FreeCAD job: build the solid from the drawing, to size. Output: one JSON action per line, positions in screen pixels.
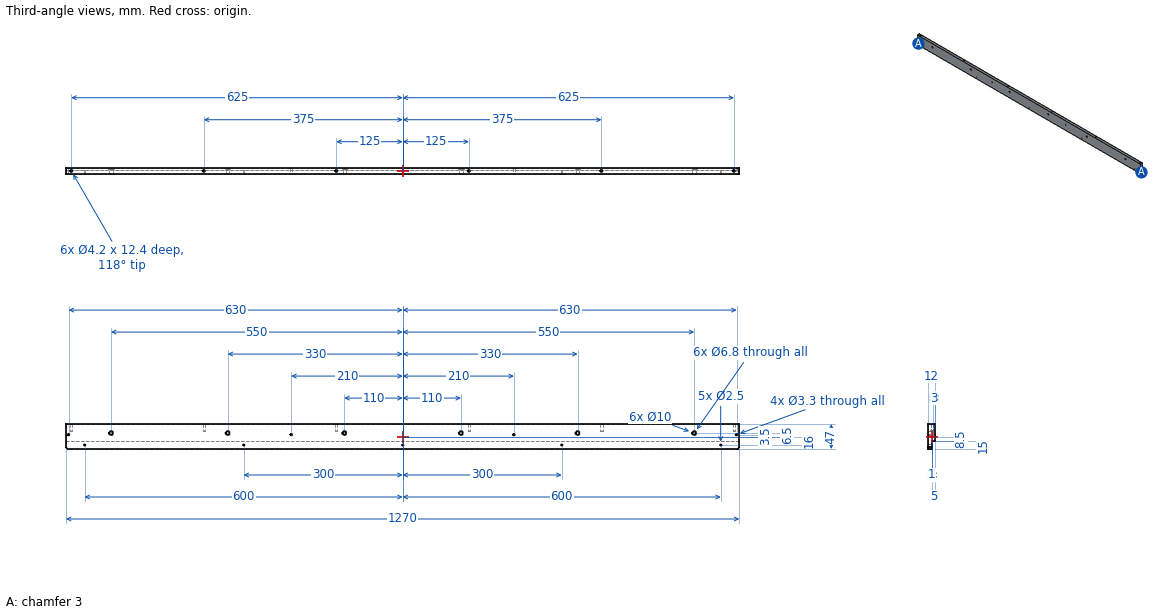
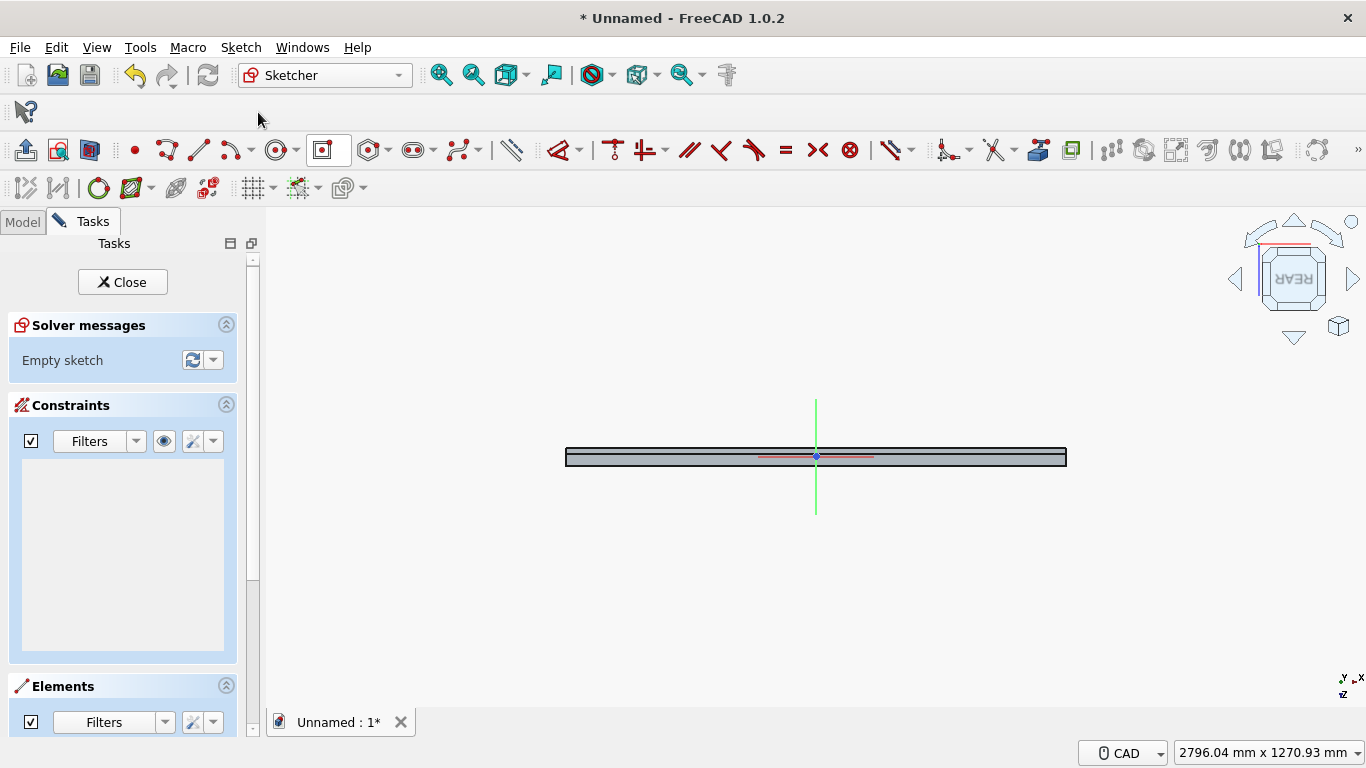
{"action": "left_click", "coordinate": [276, 150]}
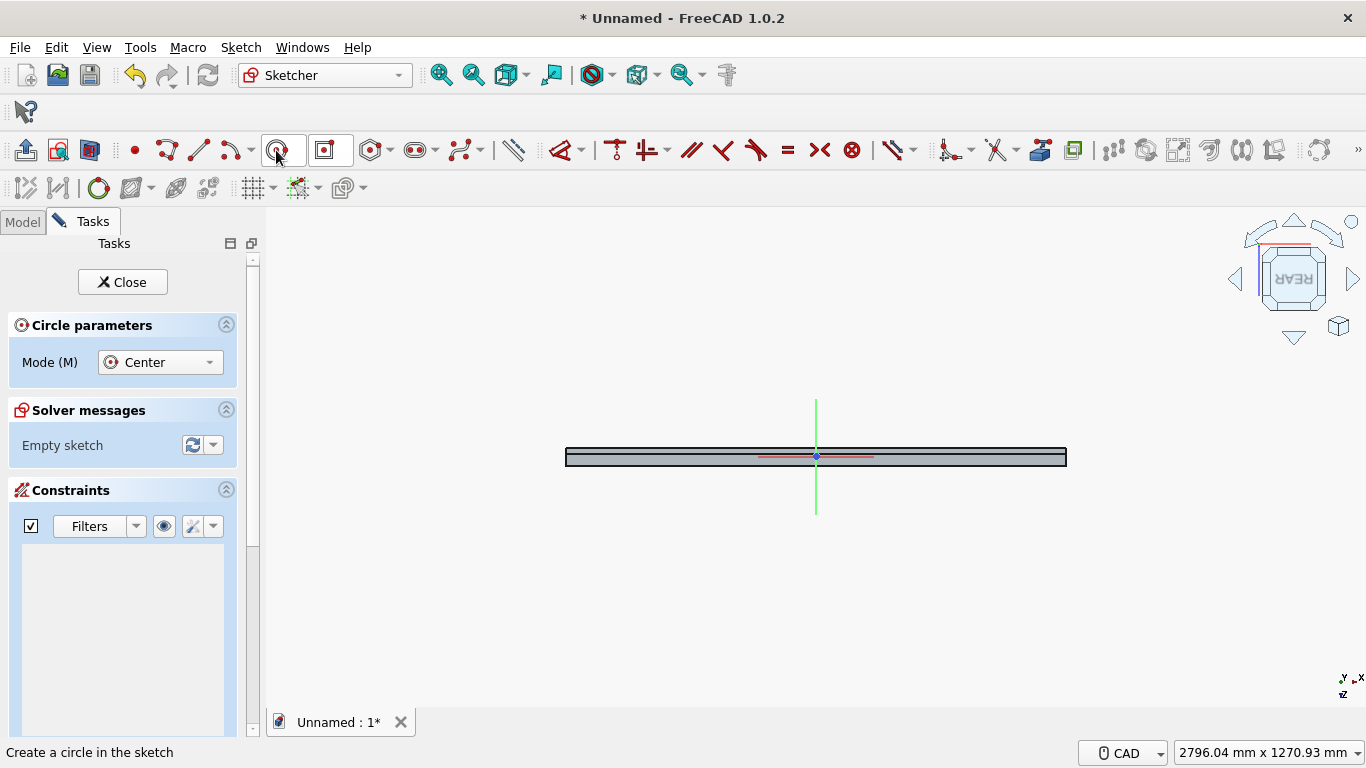
{"action": "scroll", "coordinate": [1064, 458], "scroll_direction": "up", "scroll_amount": 18}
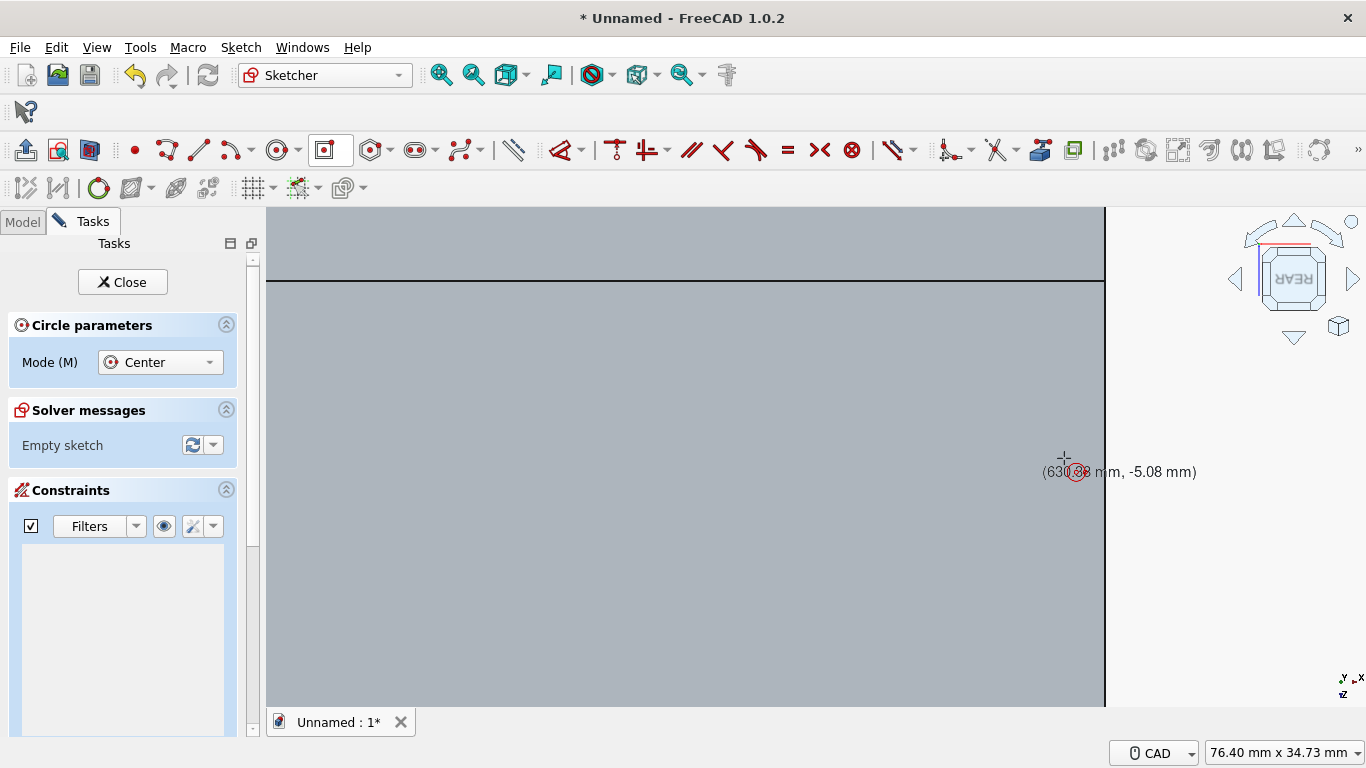
{"action": "scroll", "coordinate": [1121, 458], "scroll_direction": "down", "scroll_amount": 16}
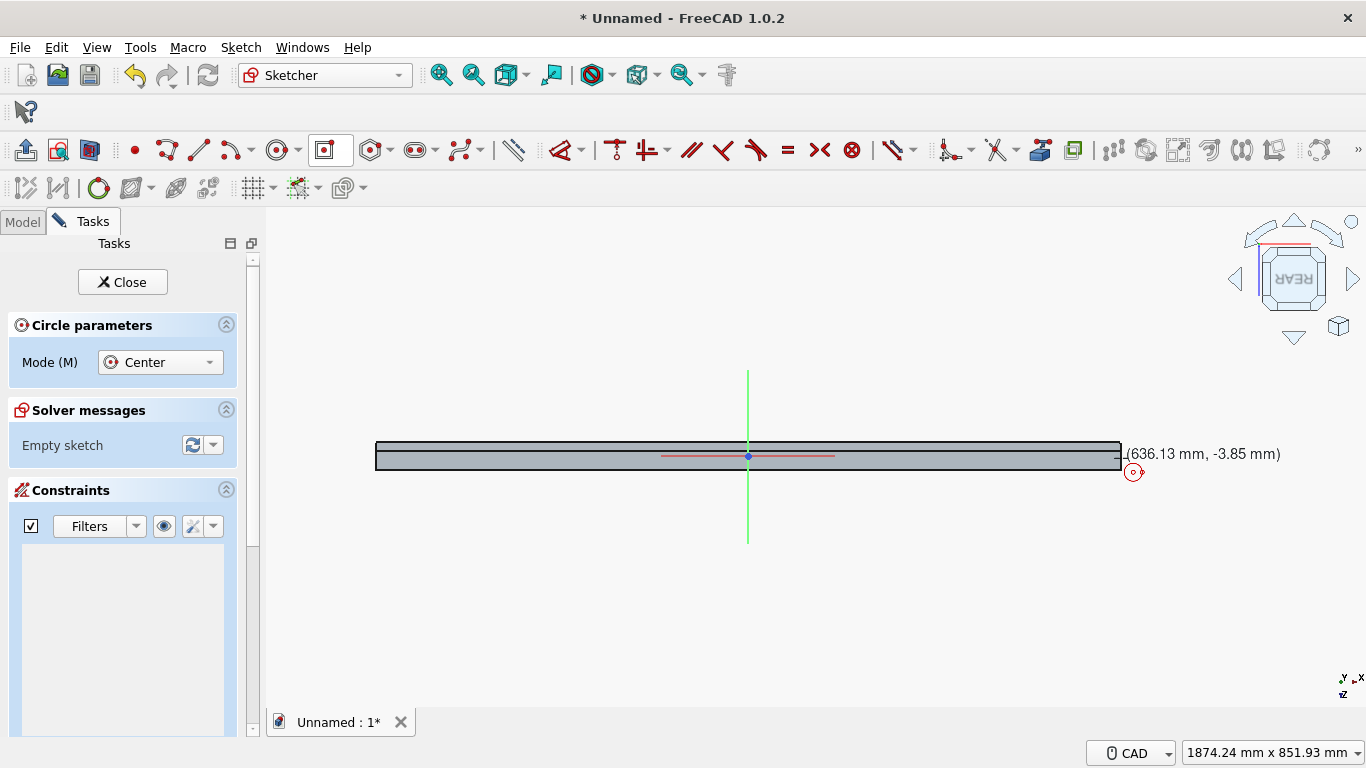
{"action": "scroll", "coordinate": [1118, 458], "scroll_direction": "up", "scroll_amount": 11}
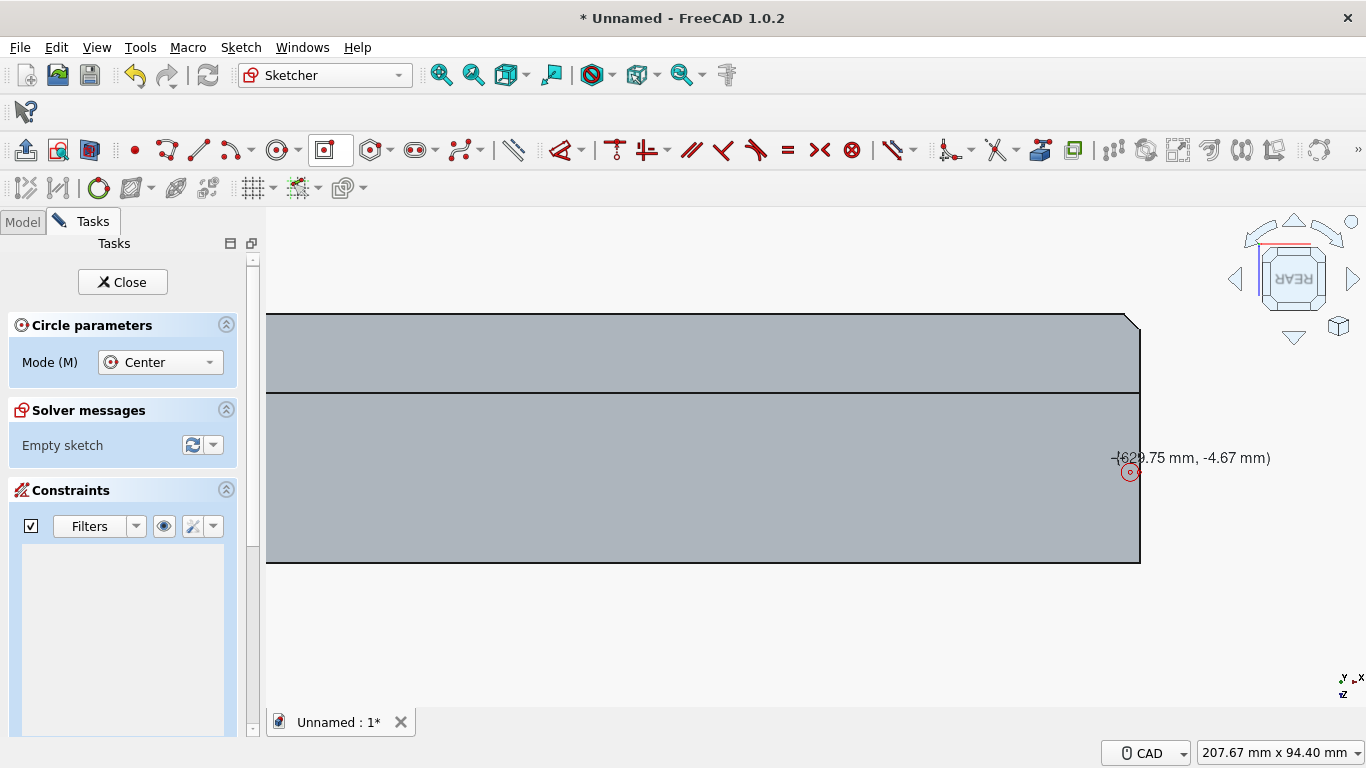
{"action": "left_click", "coordinate": [1113, 457]}
{"action": "mouse_move", "coordinate": [1119, 463]}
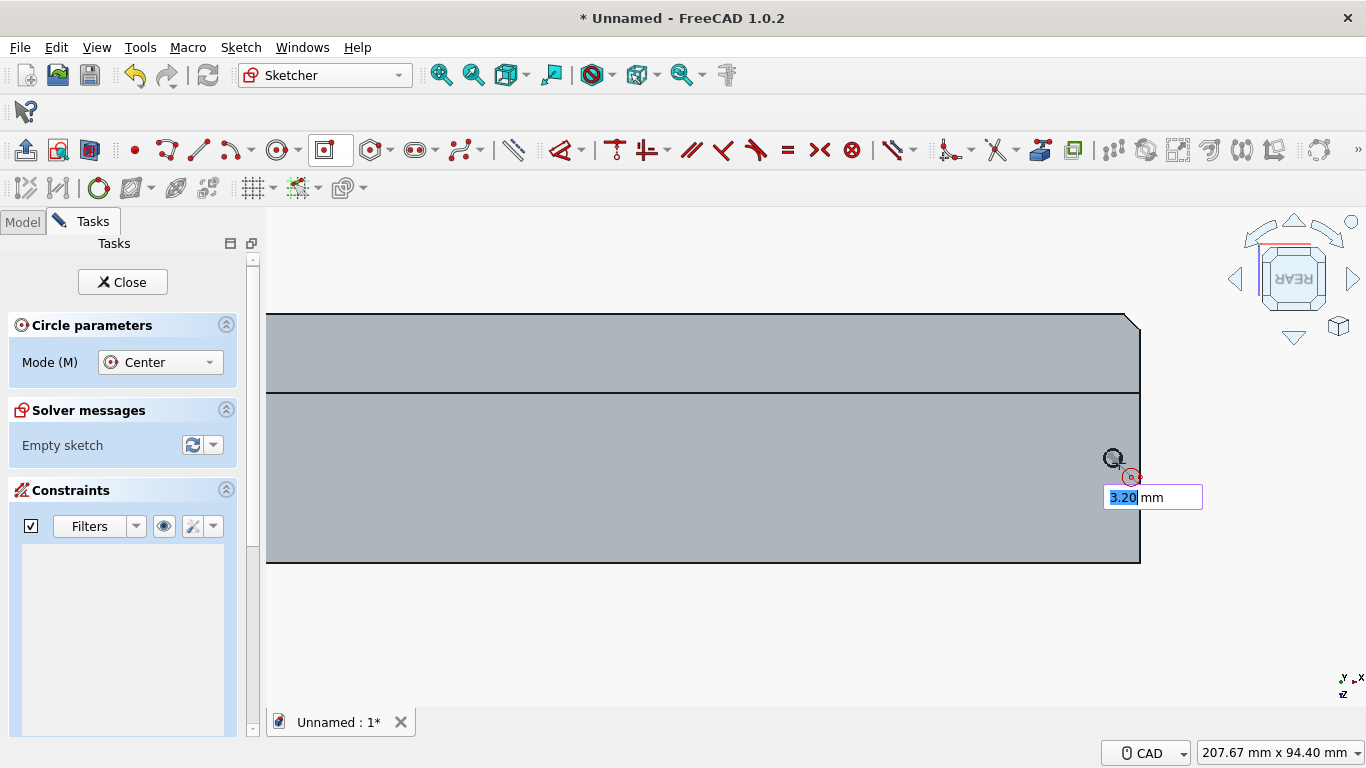
{"action": "type", "text": "3.3"}
{"action": "key", "text": "Return"}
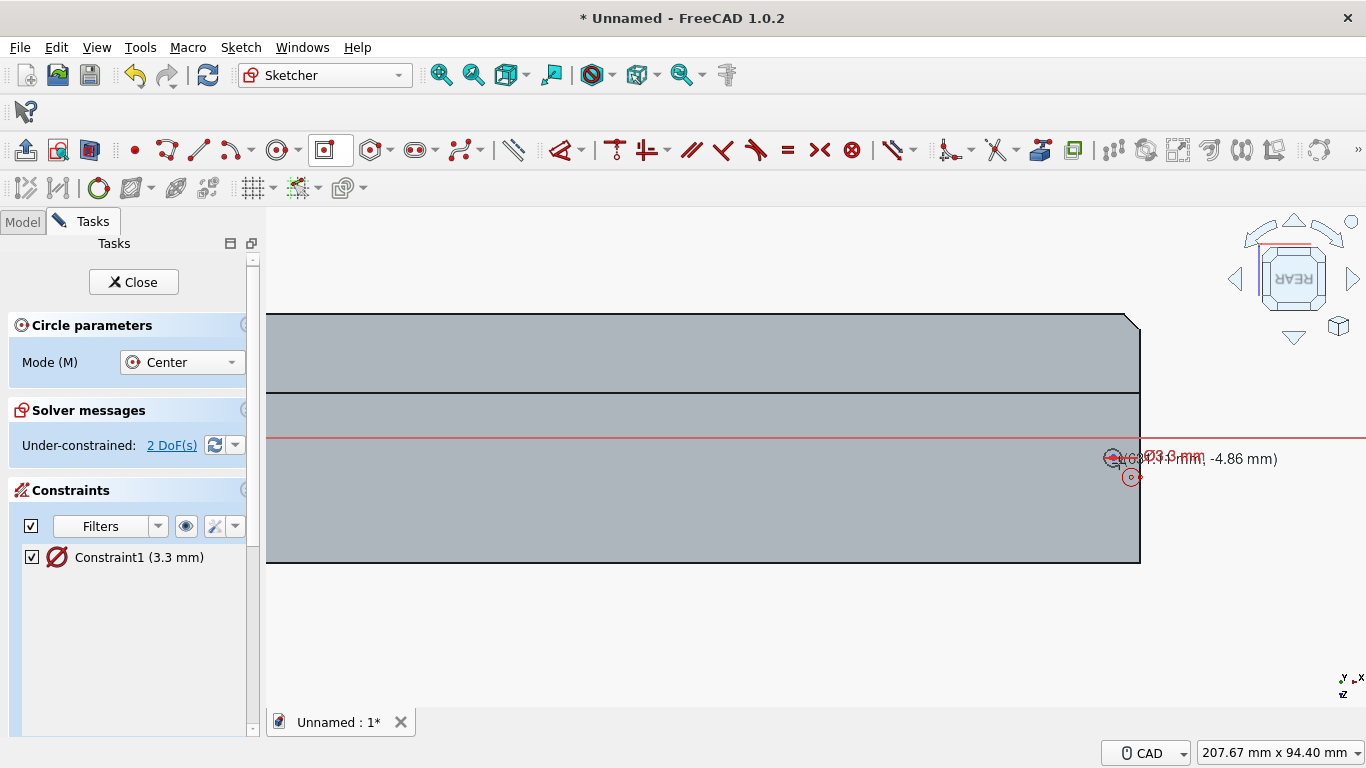
{"action": "scroll", "coordinate": [1044, 458], "scroll_direction": "down", "scroll_amount": 12}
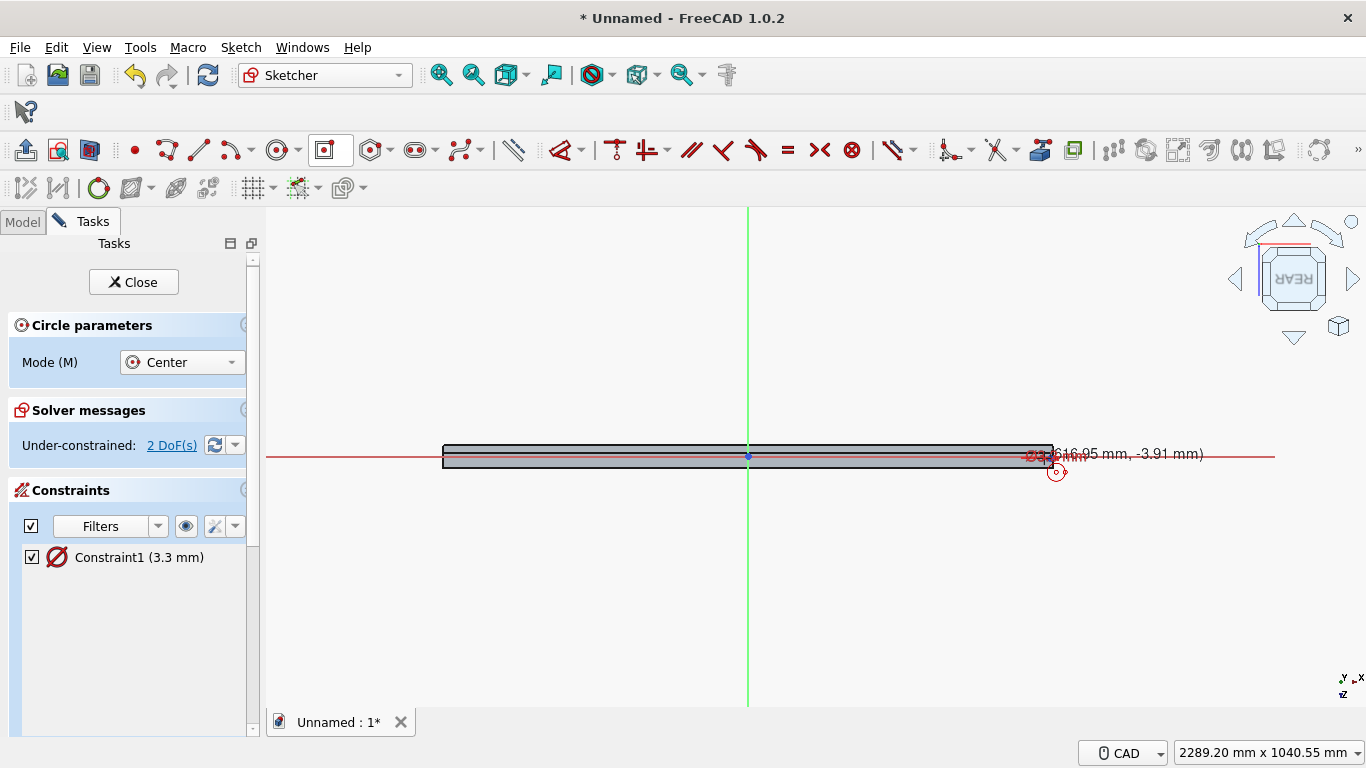
{"action": "scroll", "coordinate": [445, 458], "scroll_direction": "up", "scroll_amount": 17}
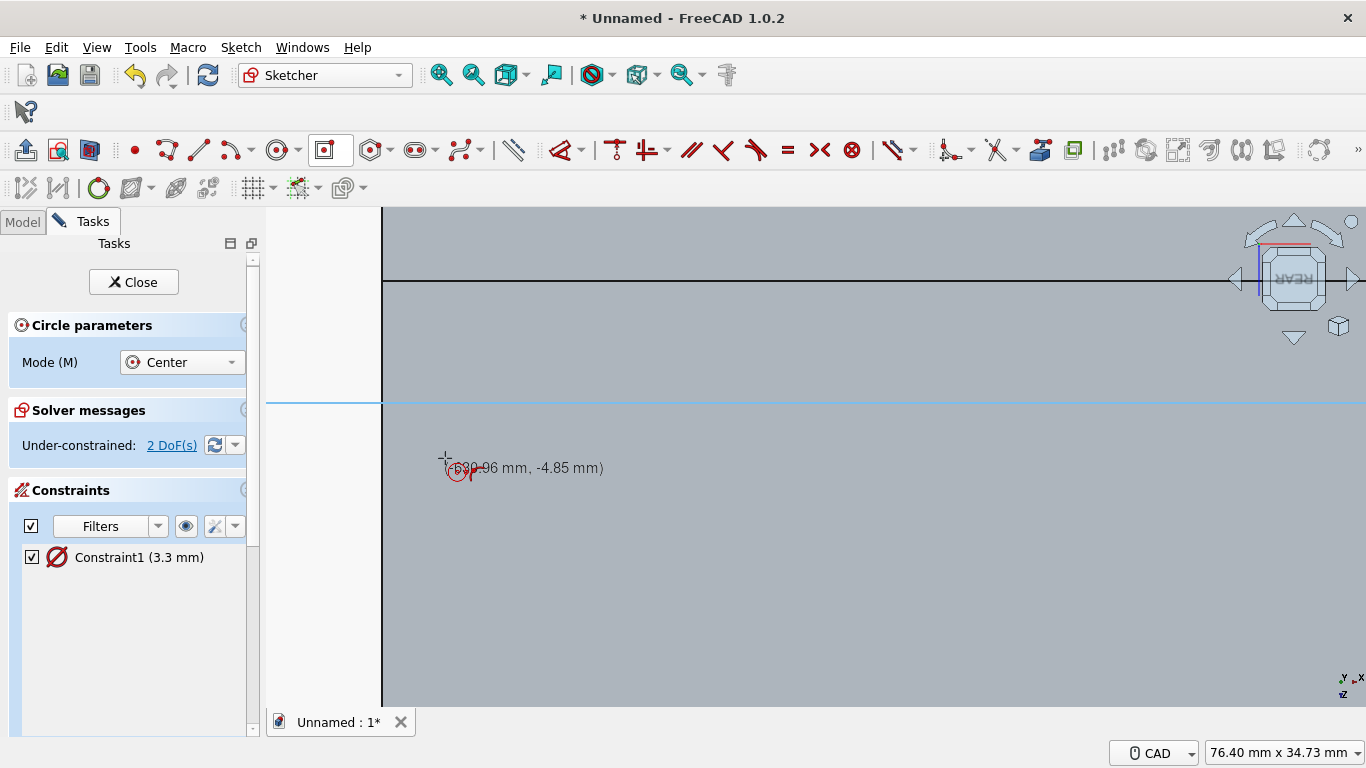
{"action": "scroll", "coordinate": [375, 458], "scroll_direction": "down", "scroll_amount": 16}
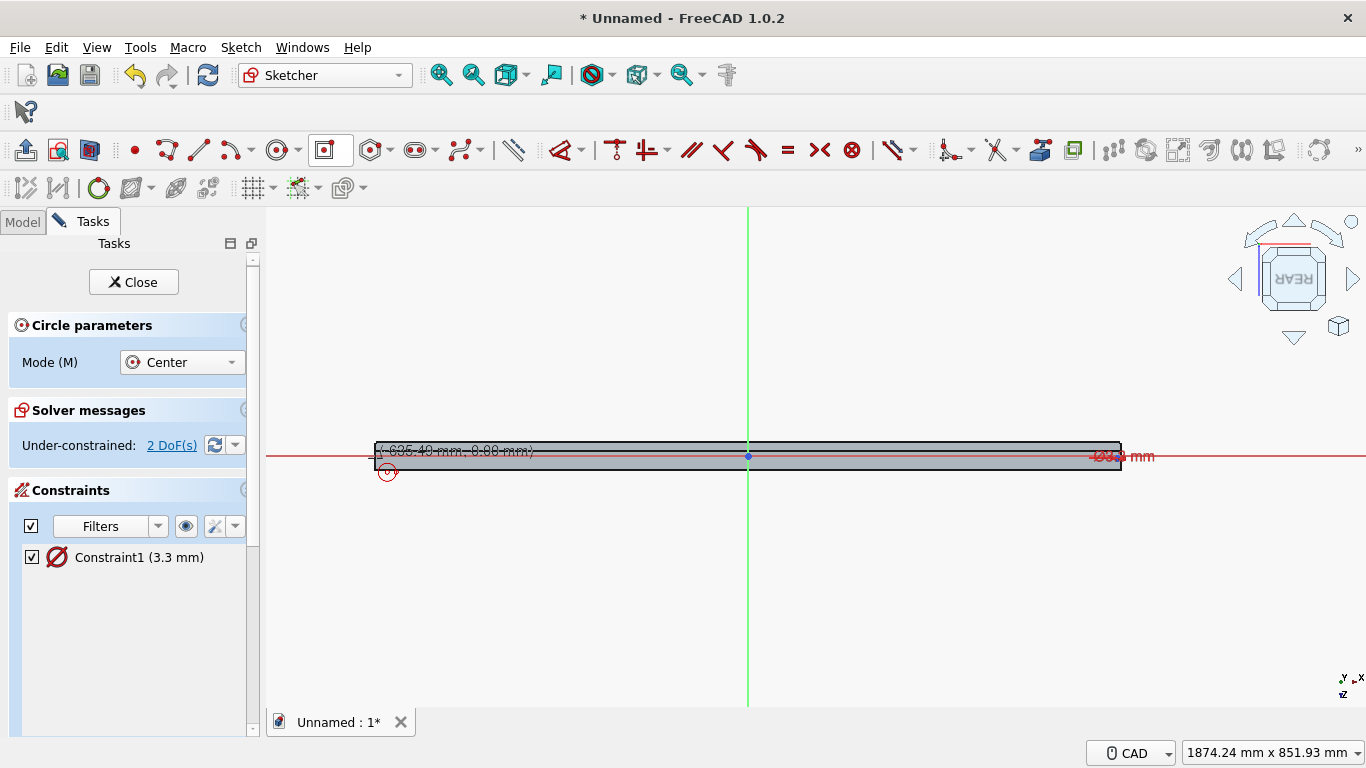
{"action": "scroll", "coordinate": [378, 458], "scroll_direction": "up", "scroll_amount": 11}